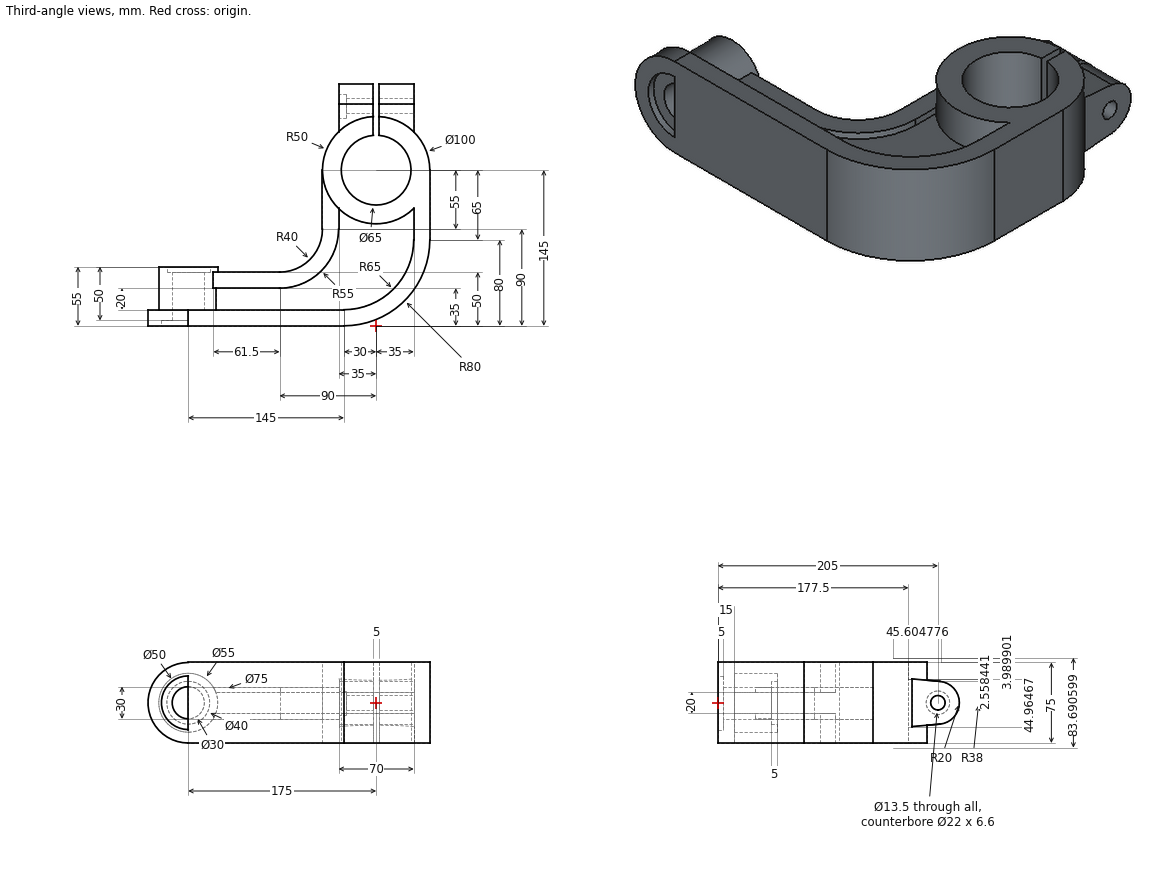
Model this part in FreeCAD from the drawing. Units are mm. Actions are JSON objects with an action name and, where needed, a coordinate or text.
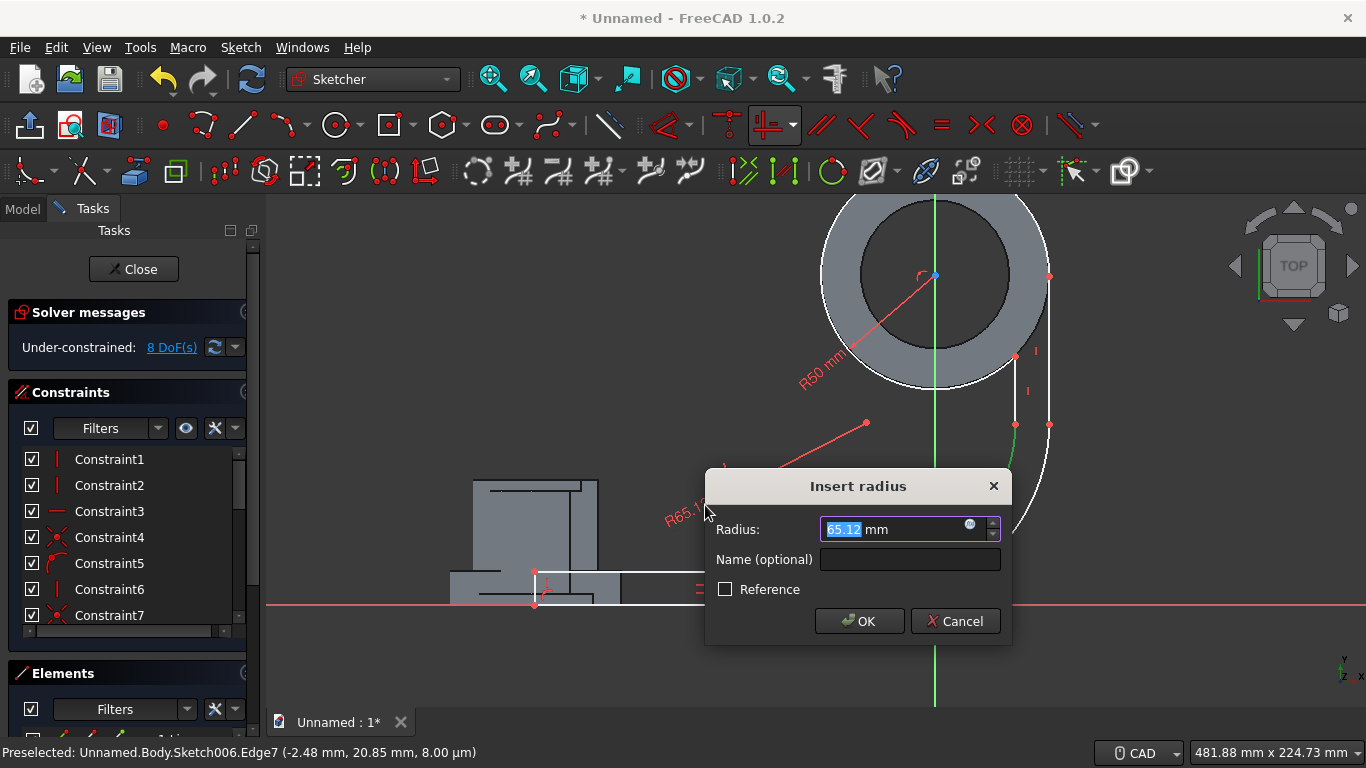
{"action": "type", "text": "65"}
{"action": "key", "text": "Return"}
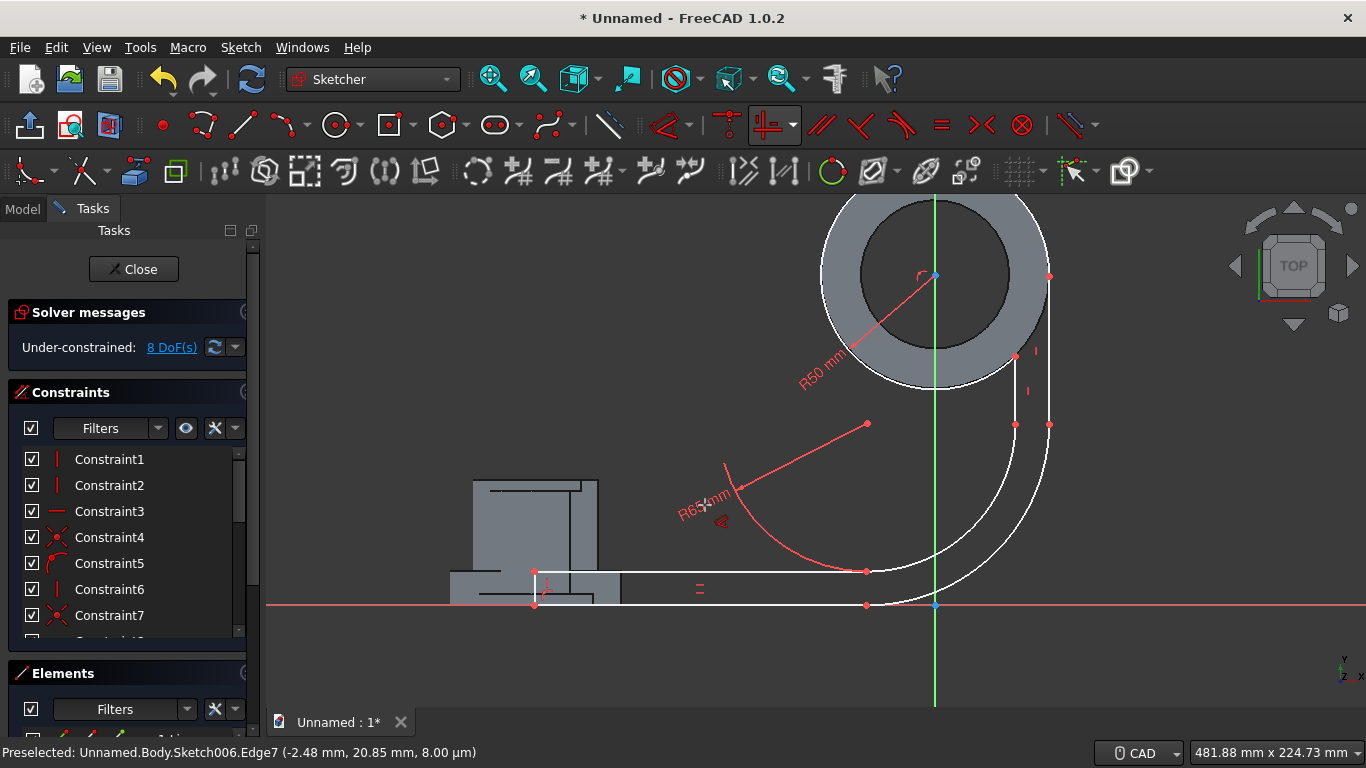
{"action": "left_click", "coordinate": [949, 586]}
{"action": "left_click", "coordinate": [860, 637]}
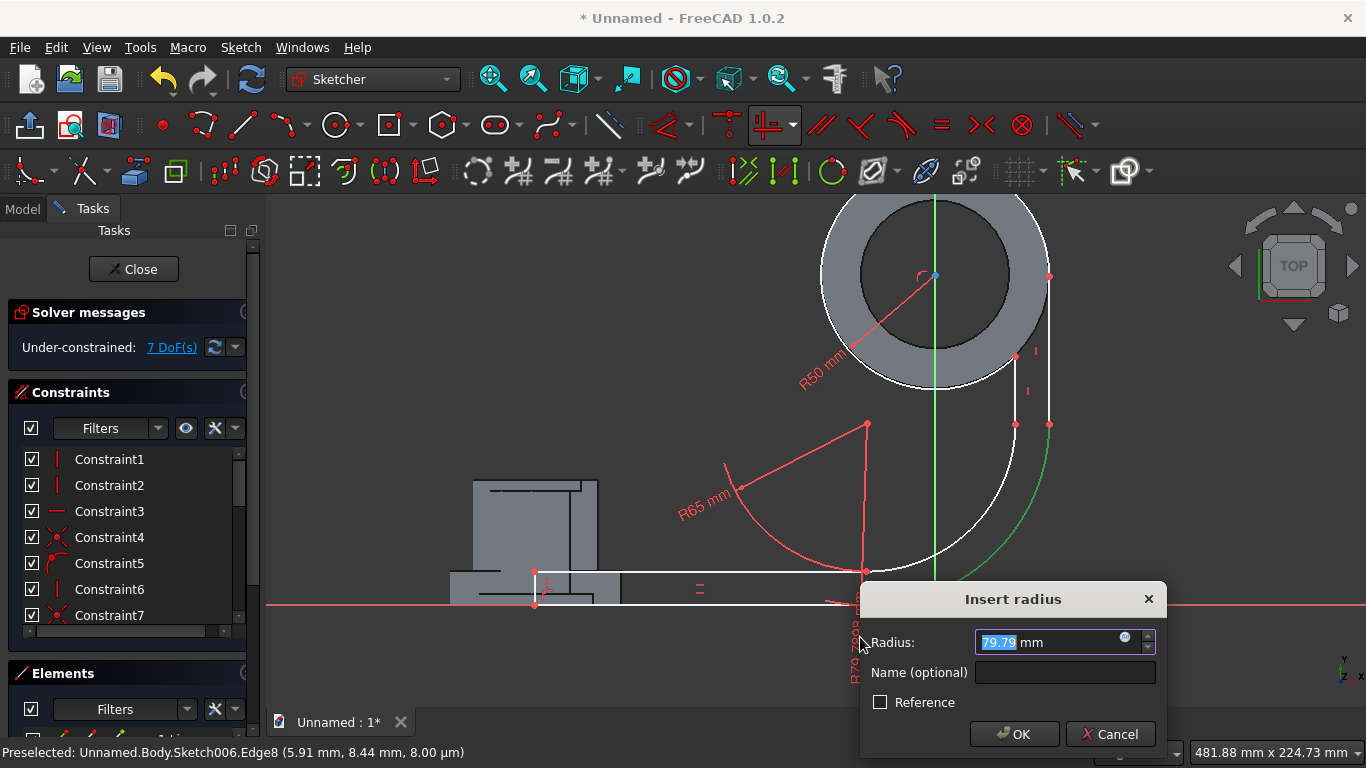
{"action": "type", "text": "80"}
{"action": "key", "text": "Return"}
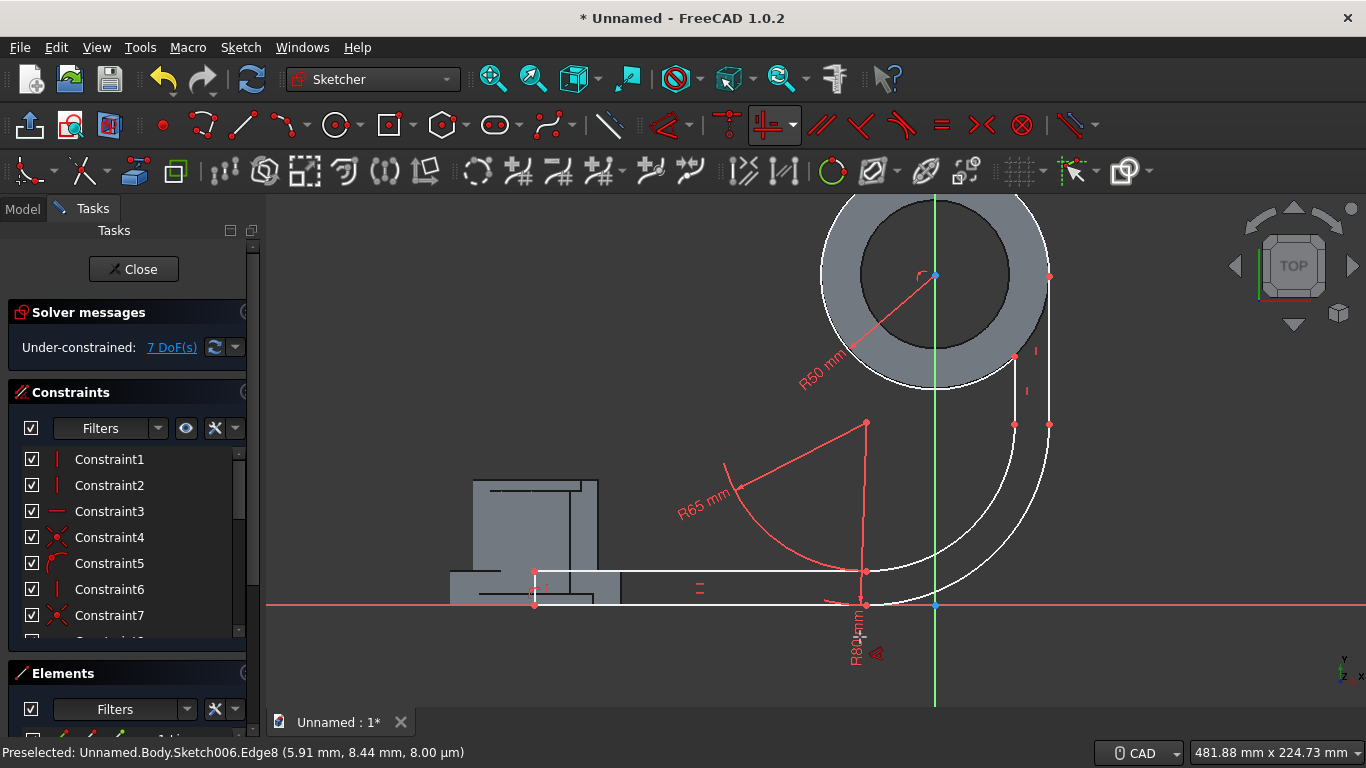
{"action": "left_click", "coordinate": [1049, 380]}
{"action": "left_click", "coordinate": [1083, 350]}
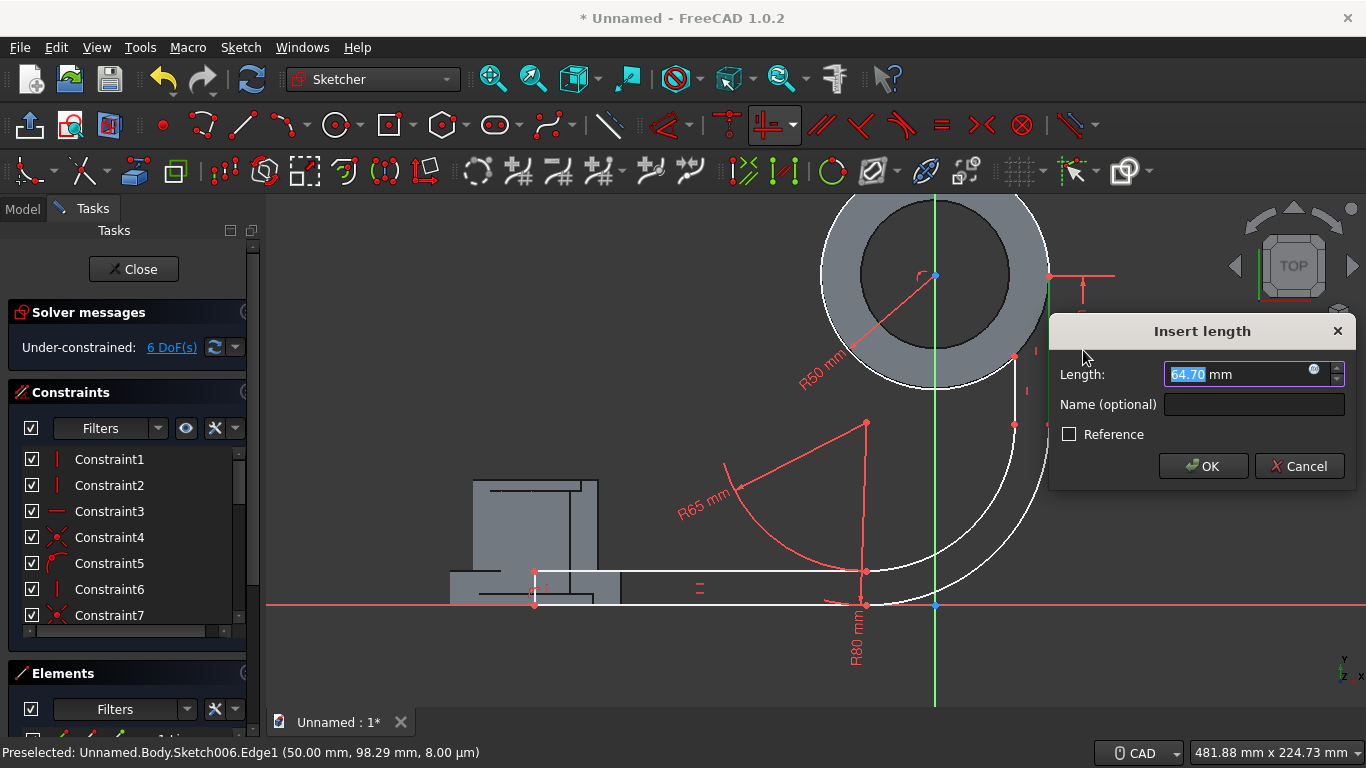
{"action": "type", "text": "65"}
{"action": "key", "text": "Return"}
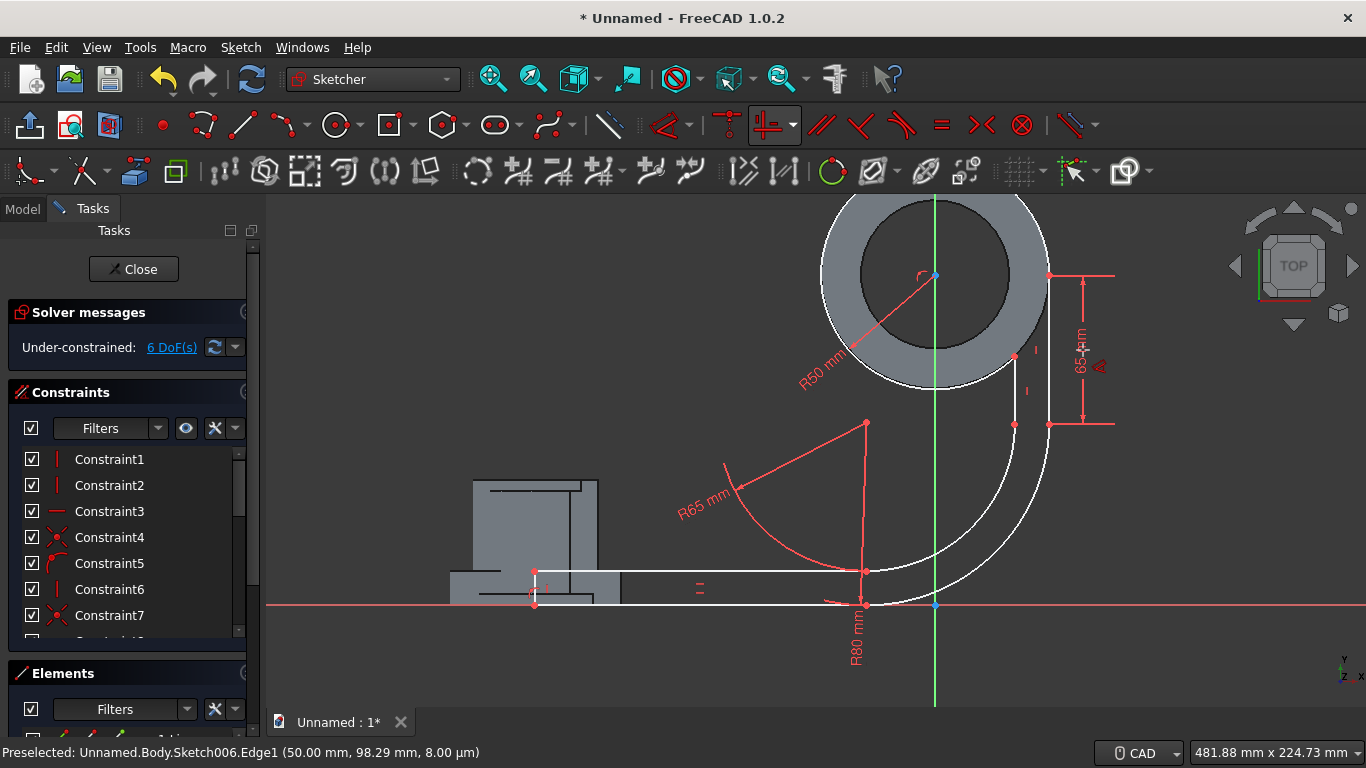
{"action": "left_click", "coordinate": [767, 571]}
{"action": "left_click", "coordinate": [701, 537]}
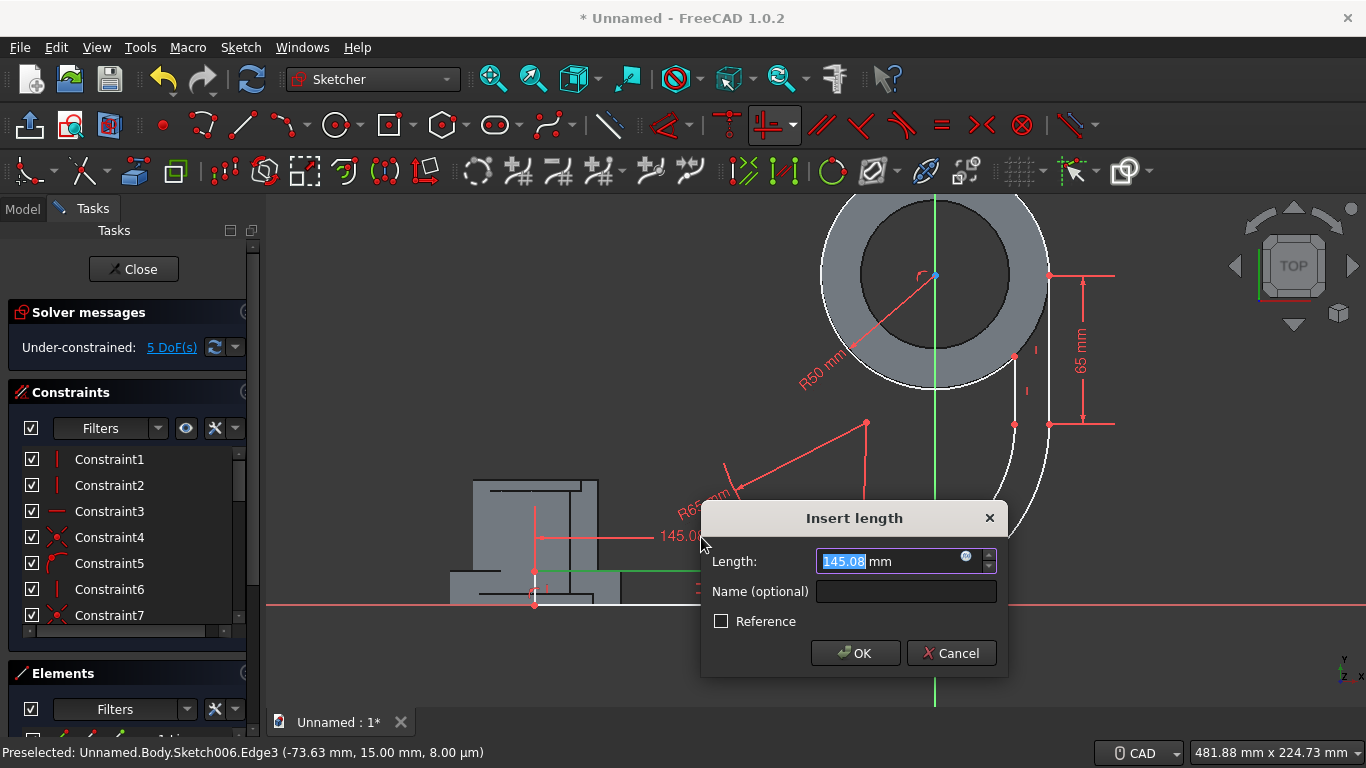
{"action": "type", "text": "145"}
{"action": "key", "text": "Return"}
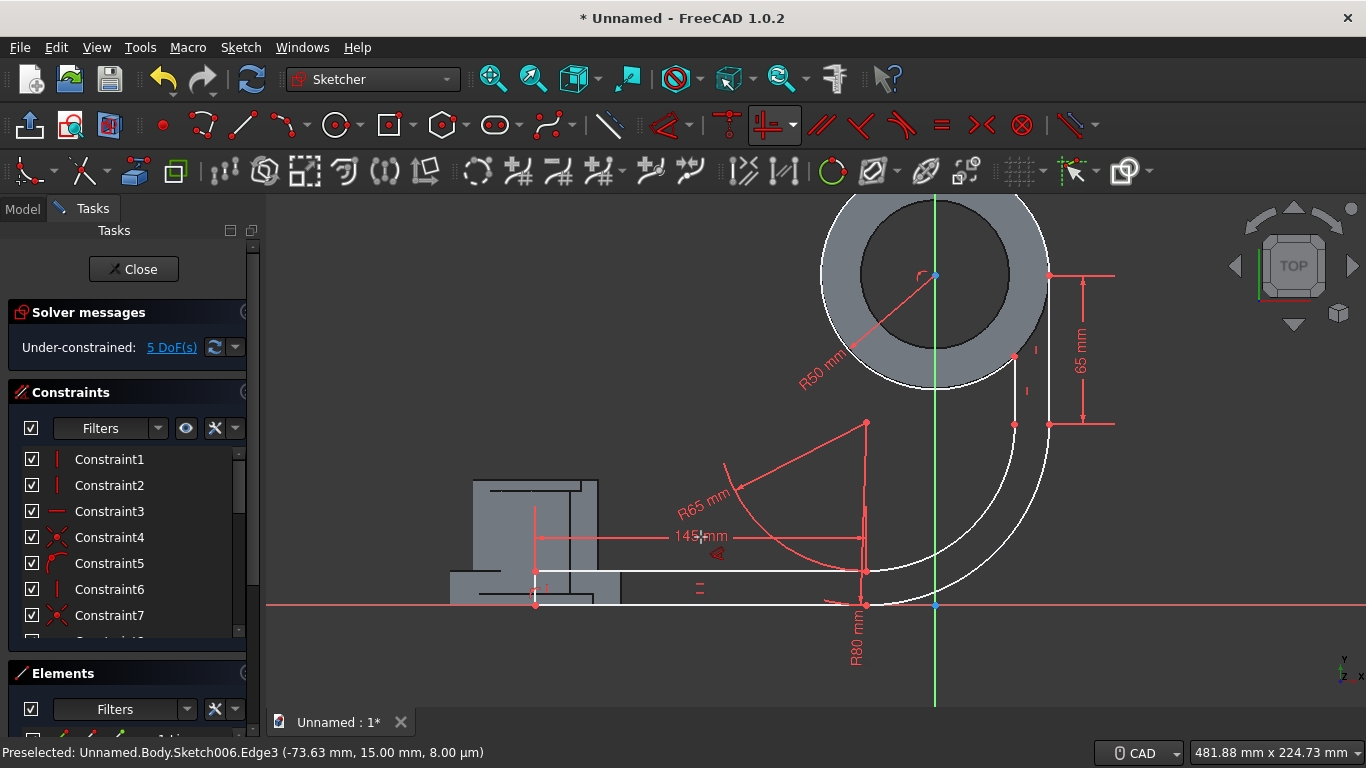
{"action": "left_click", "coordinate": [634, 605]}
{"action": "left_click", "coordinate": [701, 639]}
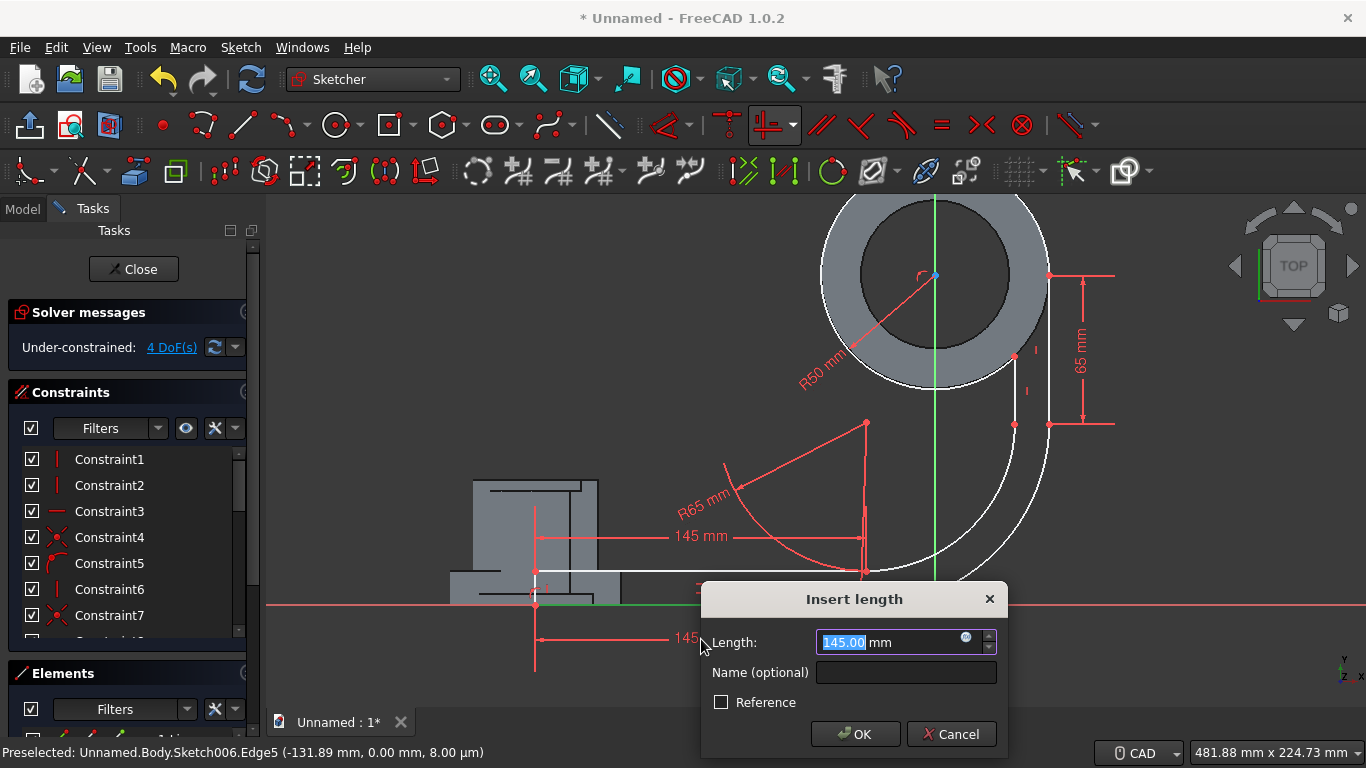
{"action": "type", "text": "145"}
{"action": "key", "text": "Return"}